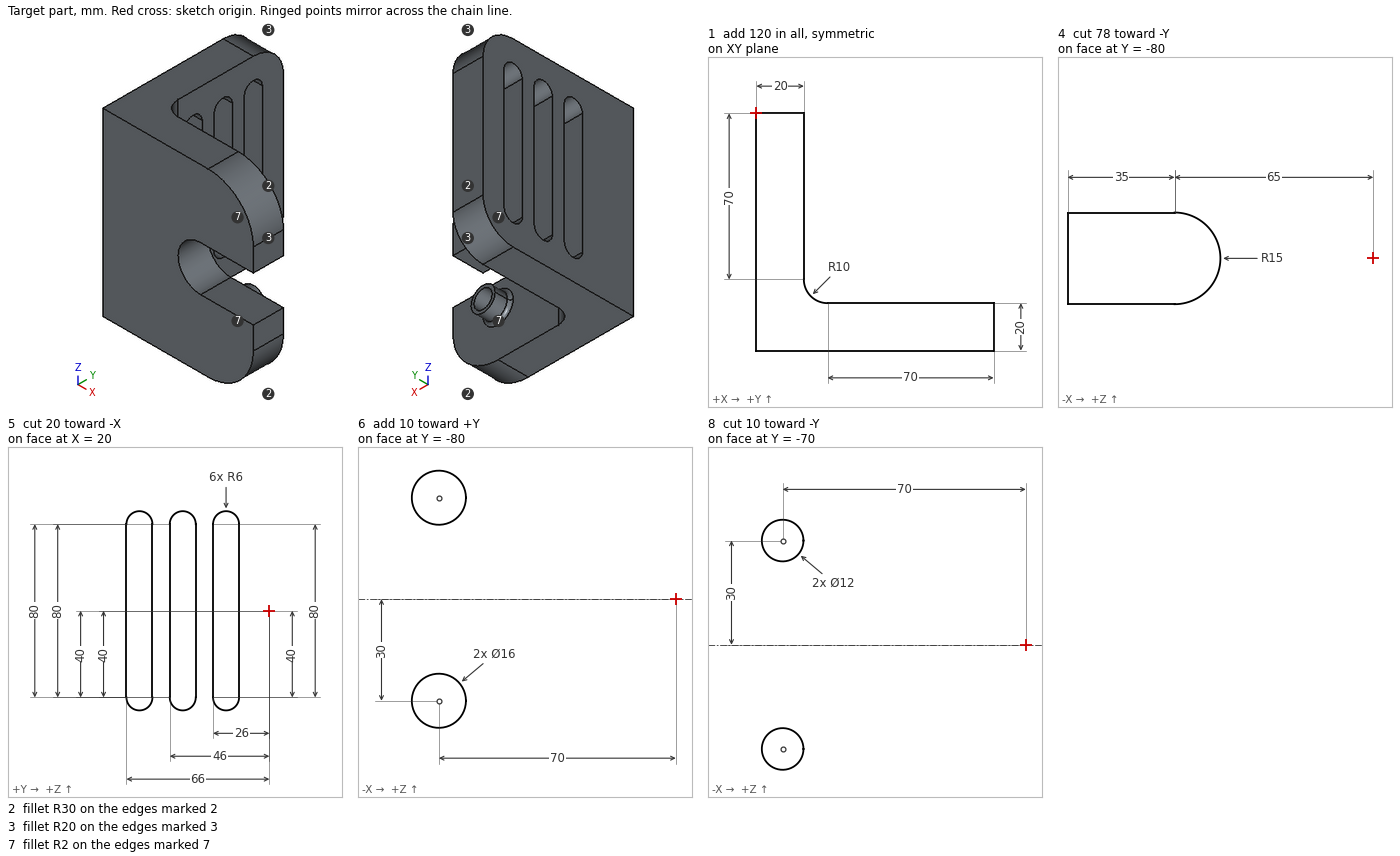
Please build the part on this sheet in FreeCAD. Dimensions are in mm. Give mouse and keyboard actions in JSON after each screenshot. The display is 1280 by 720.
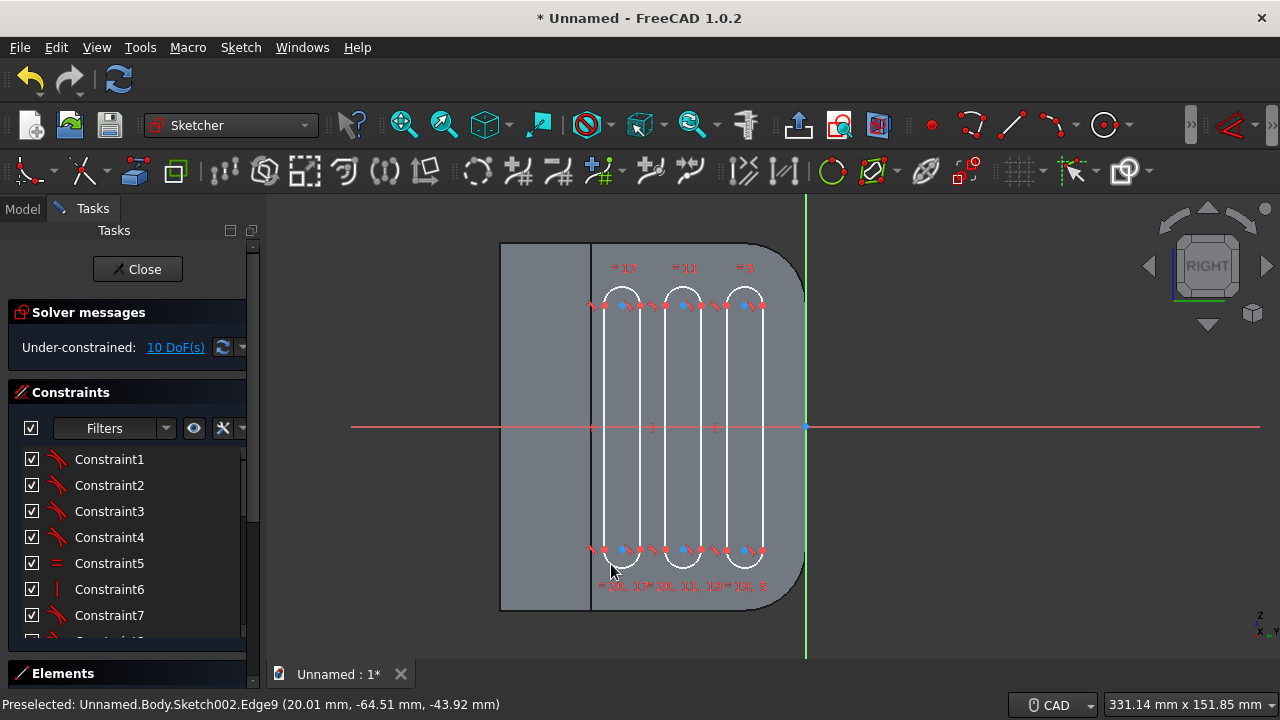
{"action": "key", "text": "d"}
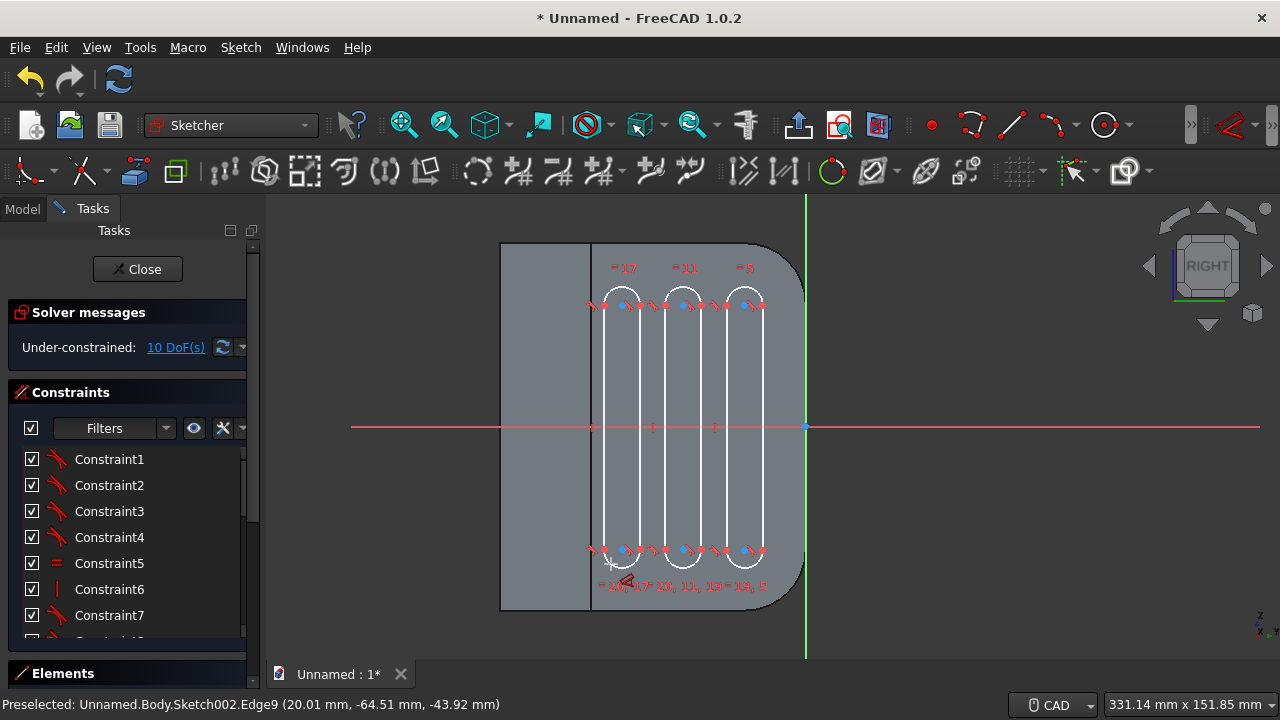
{"action": "scroll", "coordinate": [734, 565], "scroll_direction": "up", "scroll_amount": 4}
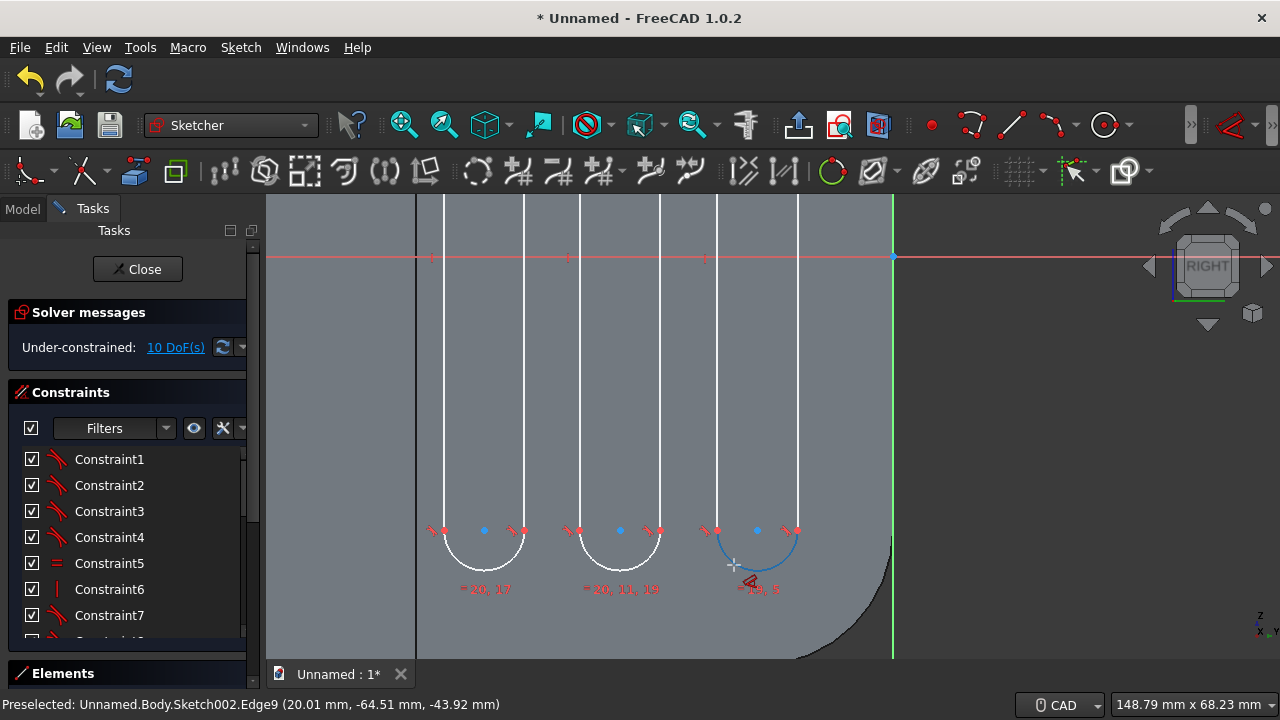
{"action": "left_click", "coordinate": [734, 563]}
{"action": "left_click", "coordinate": [715, 589]}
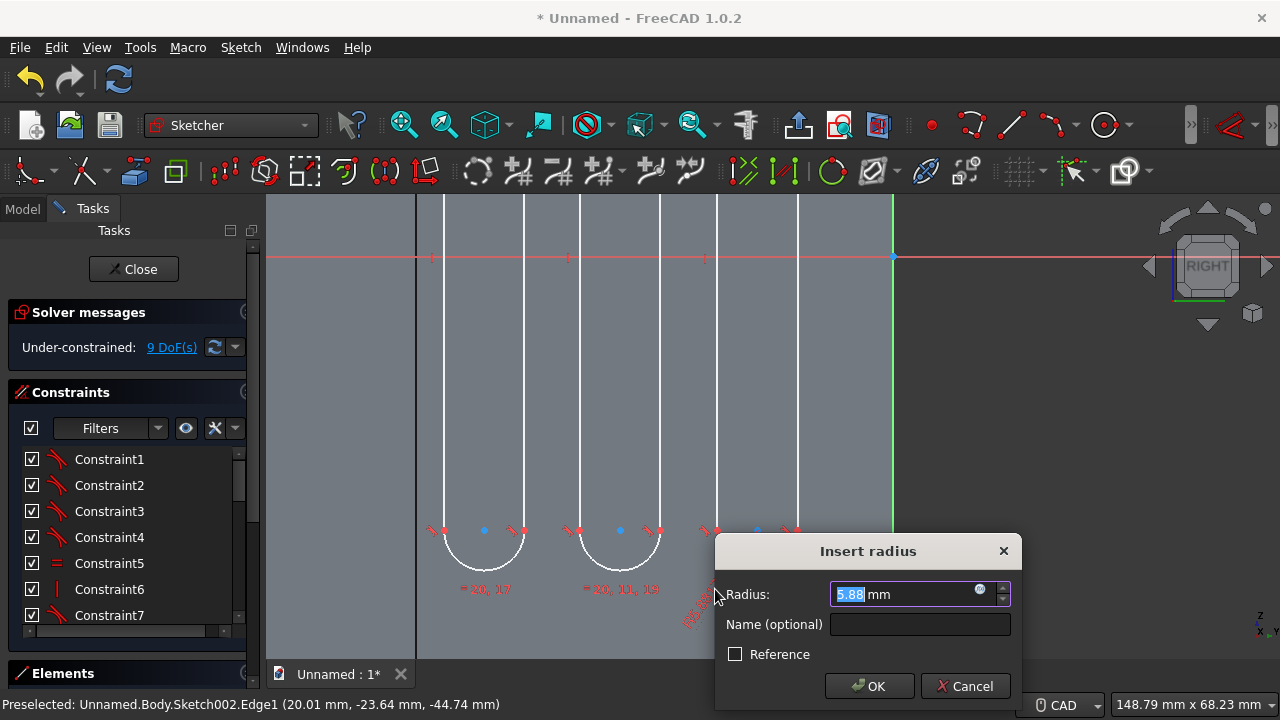
{"action": "type", "text": "6"}
{"action": "key", "text": "Return"}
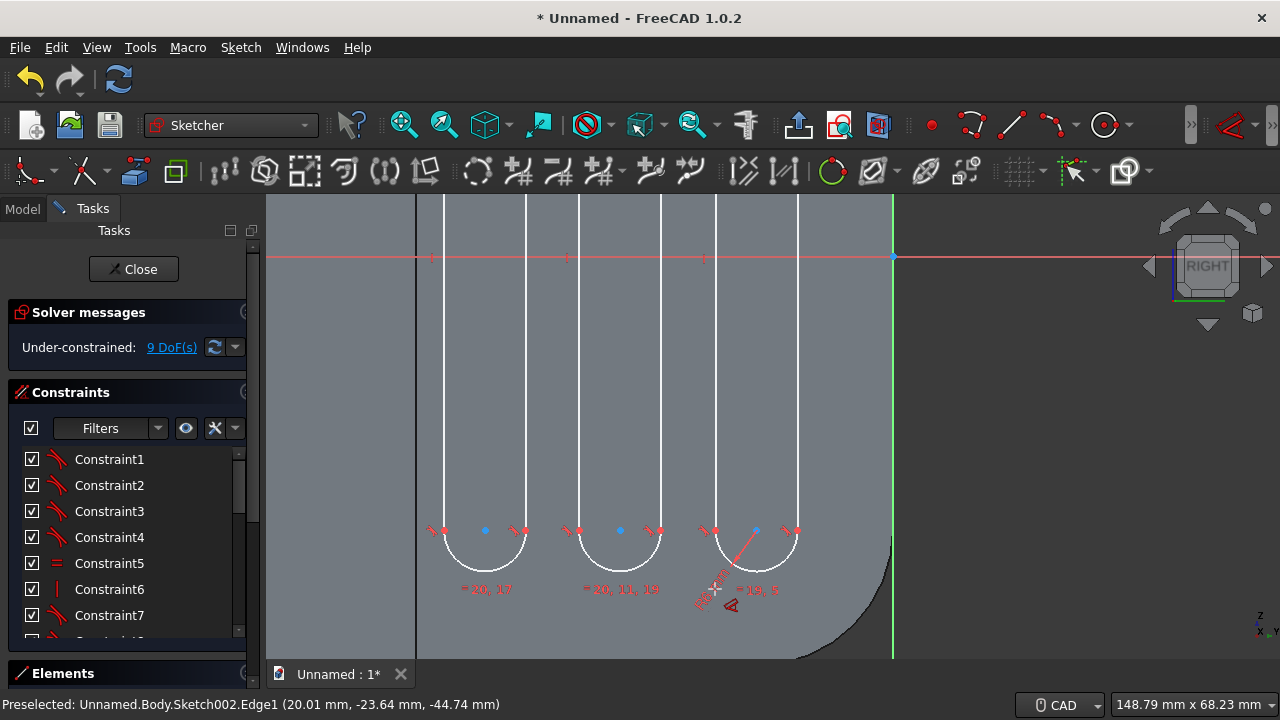
{"action": "left_click", "coordinate": [716, 367]}
{"action": "left_click", "coordinate": [750, 376]}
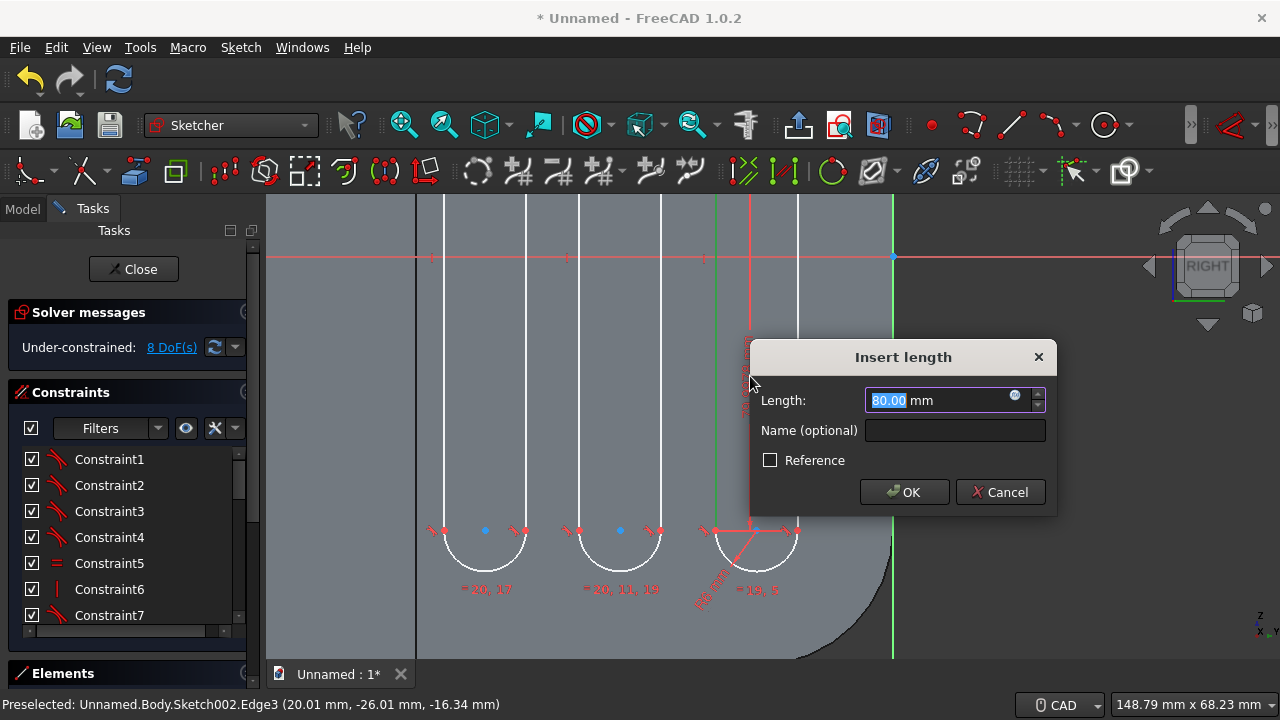
{"action": "type", "text": "80"}
{"action": "key", "text": "Return"}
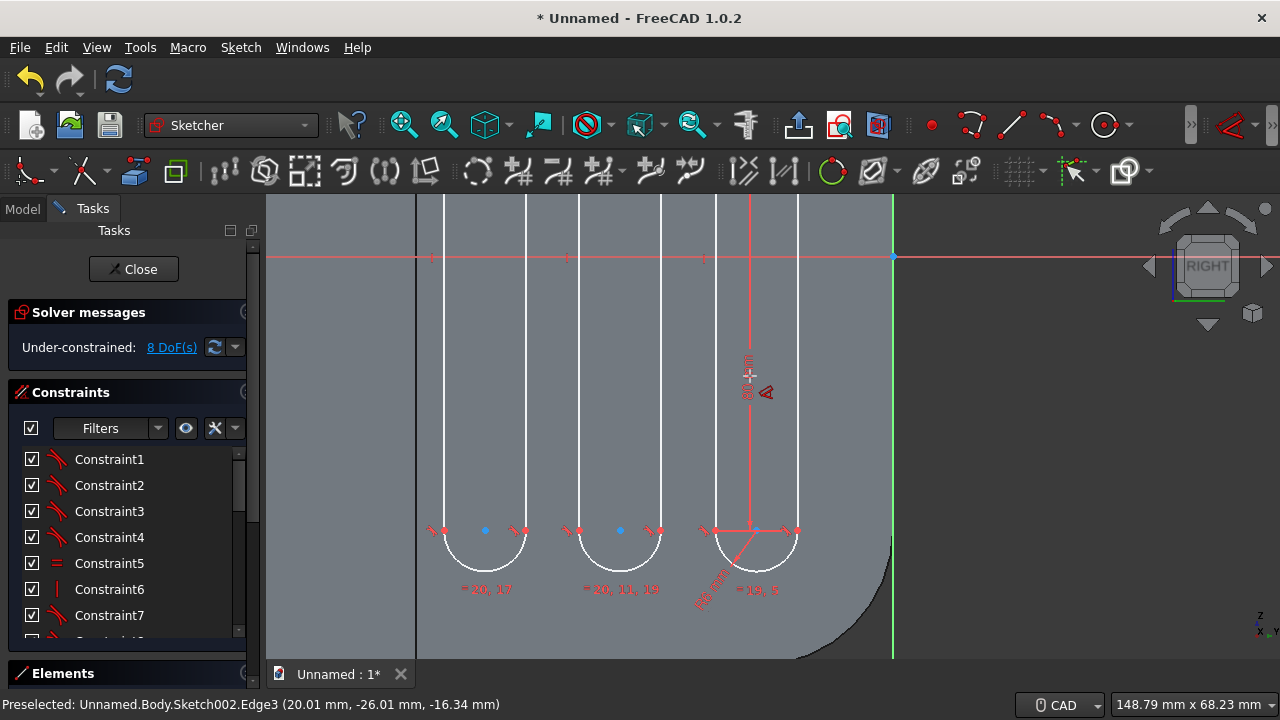
{"action": "left_click", "coordinate": [579, 367]}
{"action": "left_click", "coordinate": [545, 376]}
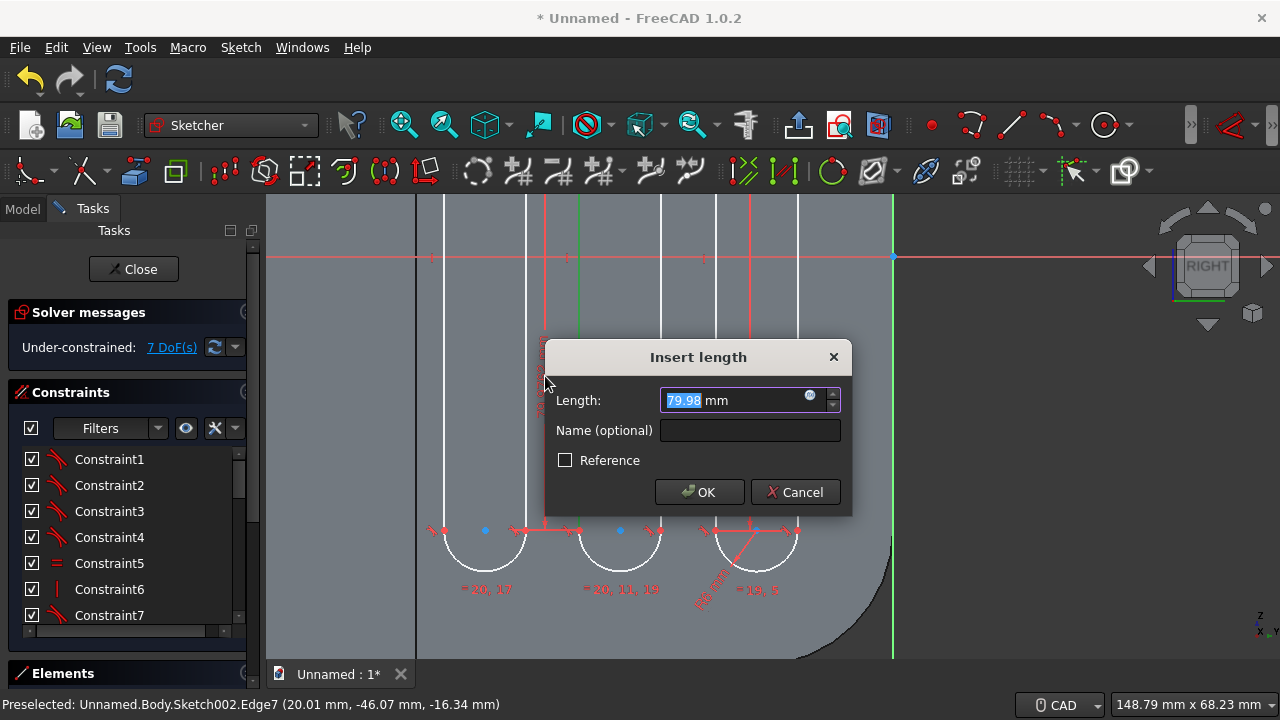
{"action": "type", "text": "80"}
{"action": "key", "text": "Return"}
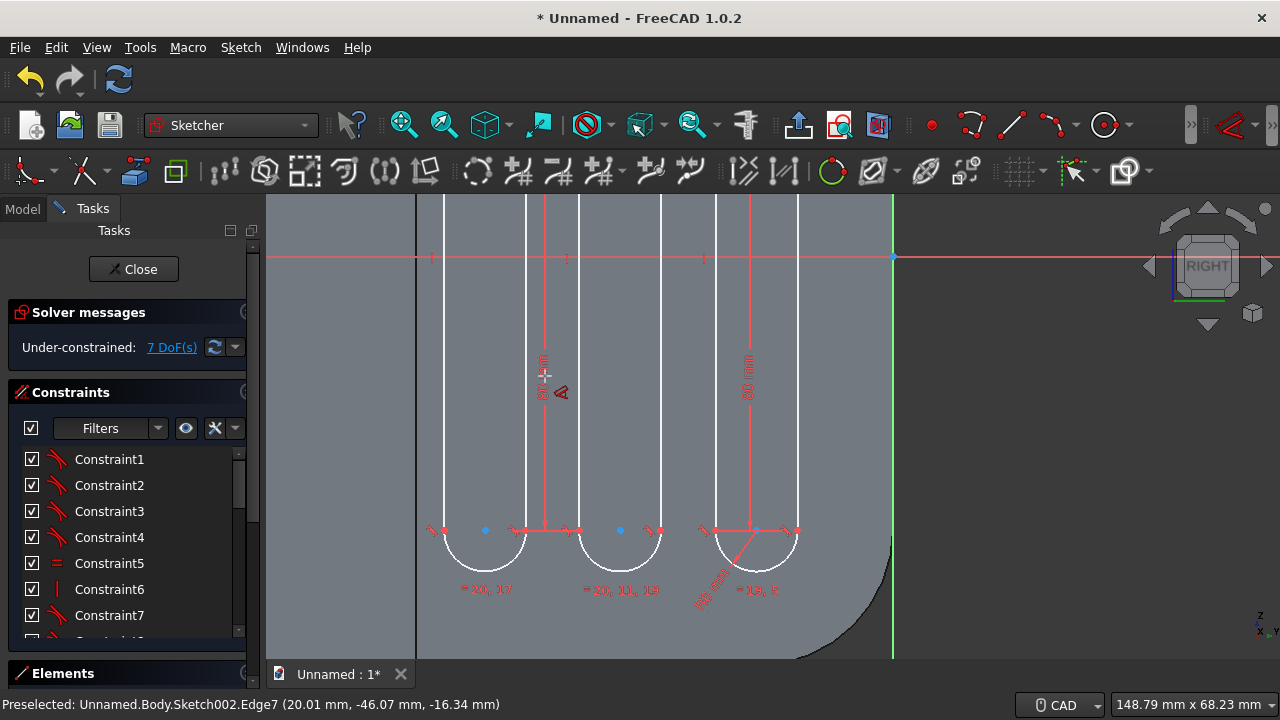
{"action": "left_click", "coordinate": [444, 367]}
{"action": "left_click", "coordinate": [410, 376]}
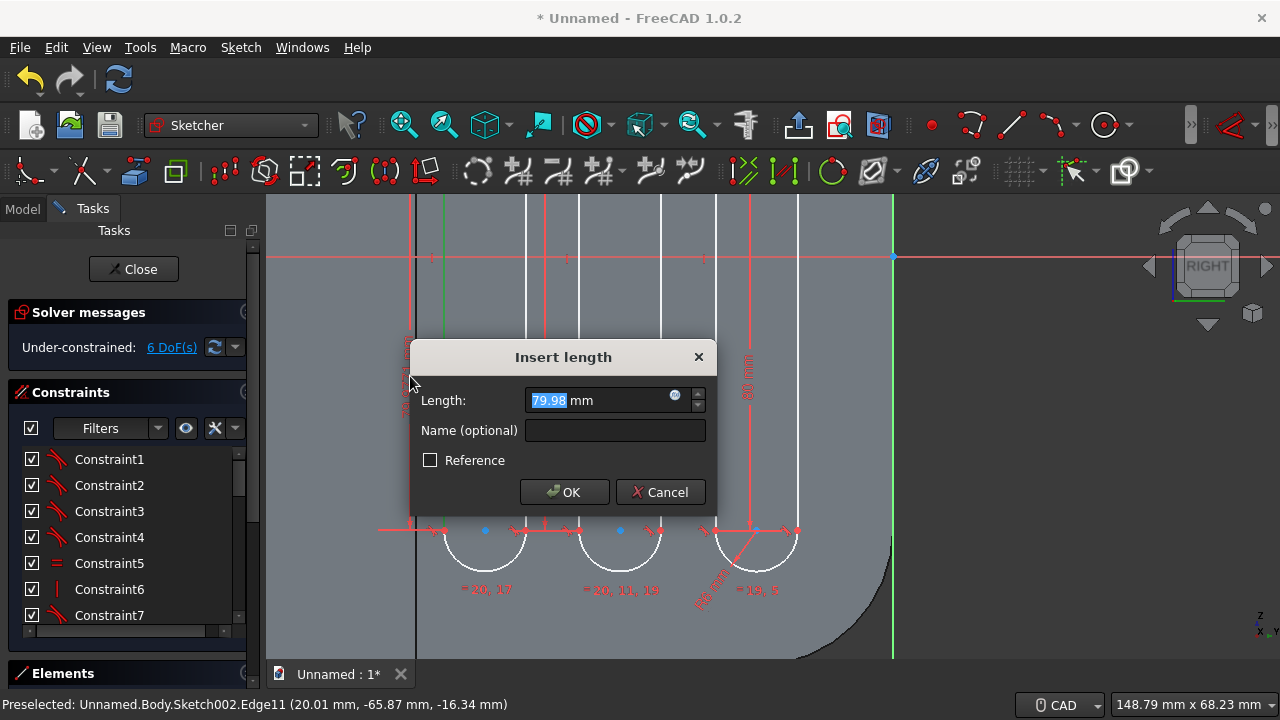
{"action": "type", "text": "80"}
{"action": "key", "text": "Return"}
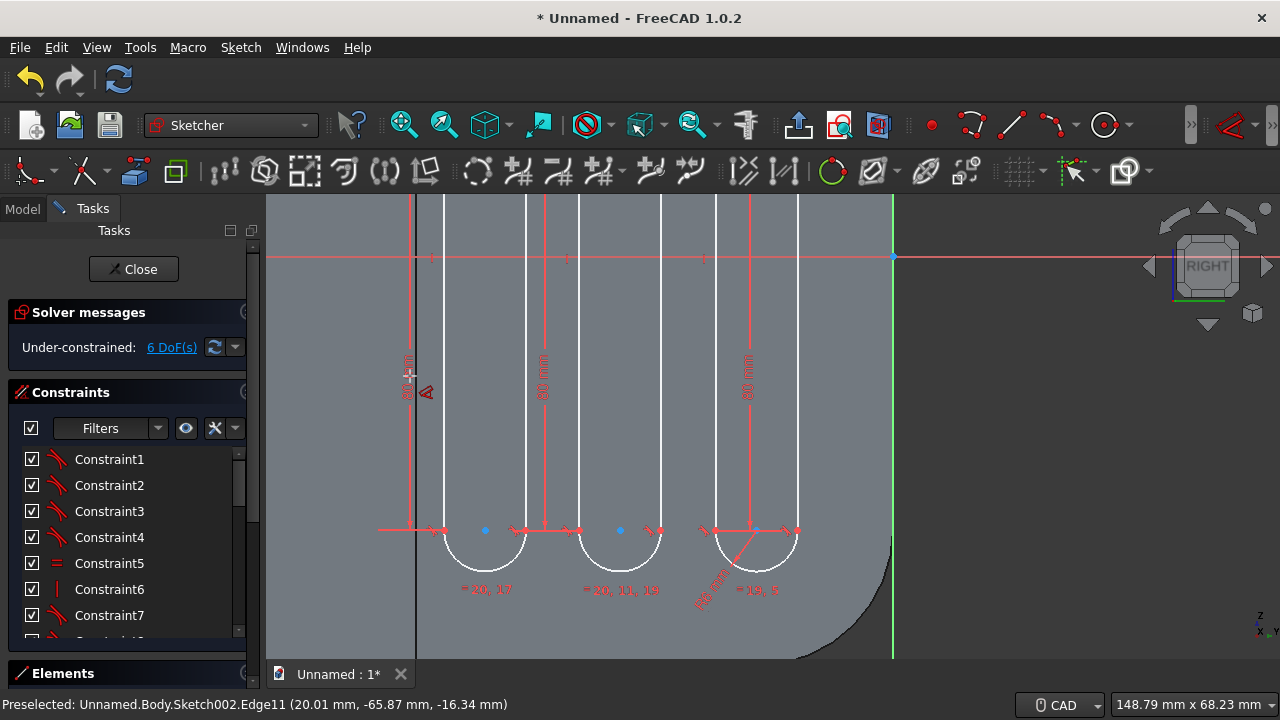
{"action": "left_click", "coordinate": [716, 531]}
{"action": "left_click", "coordinate": [804, 565]}